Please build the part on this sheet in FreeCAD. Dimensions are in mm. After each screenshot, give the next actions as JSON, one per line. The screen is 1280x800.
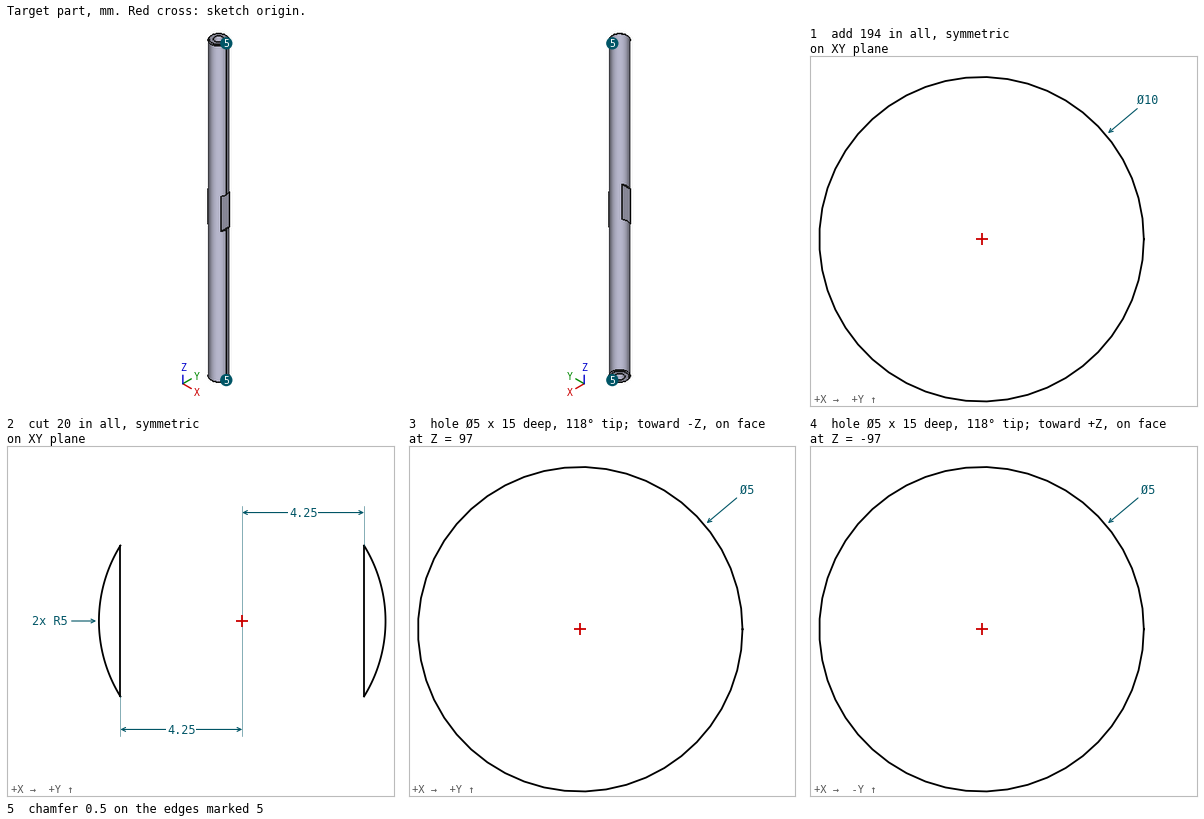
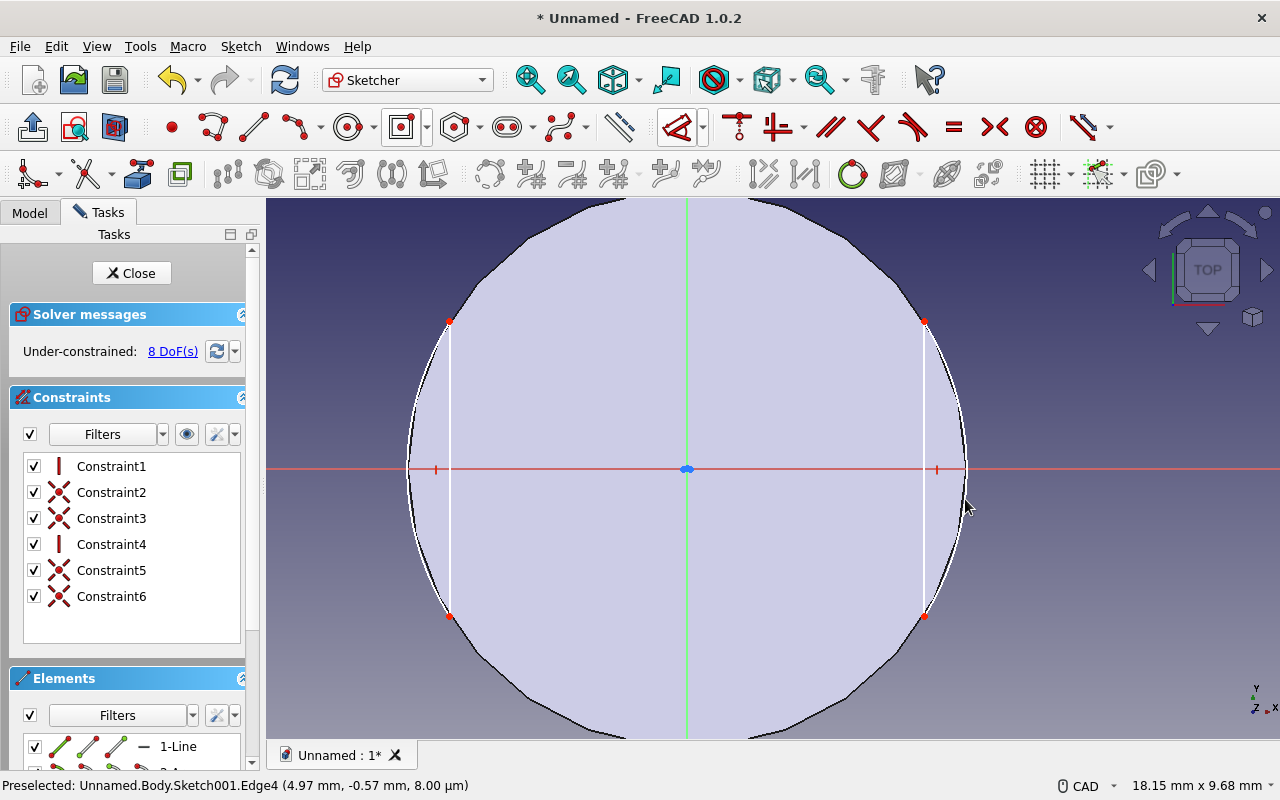
{"action": "left_click", "coordinate": [414, 408]}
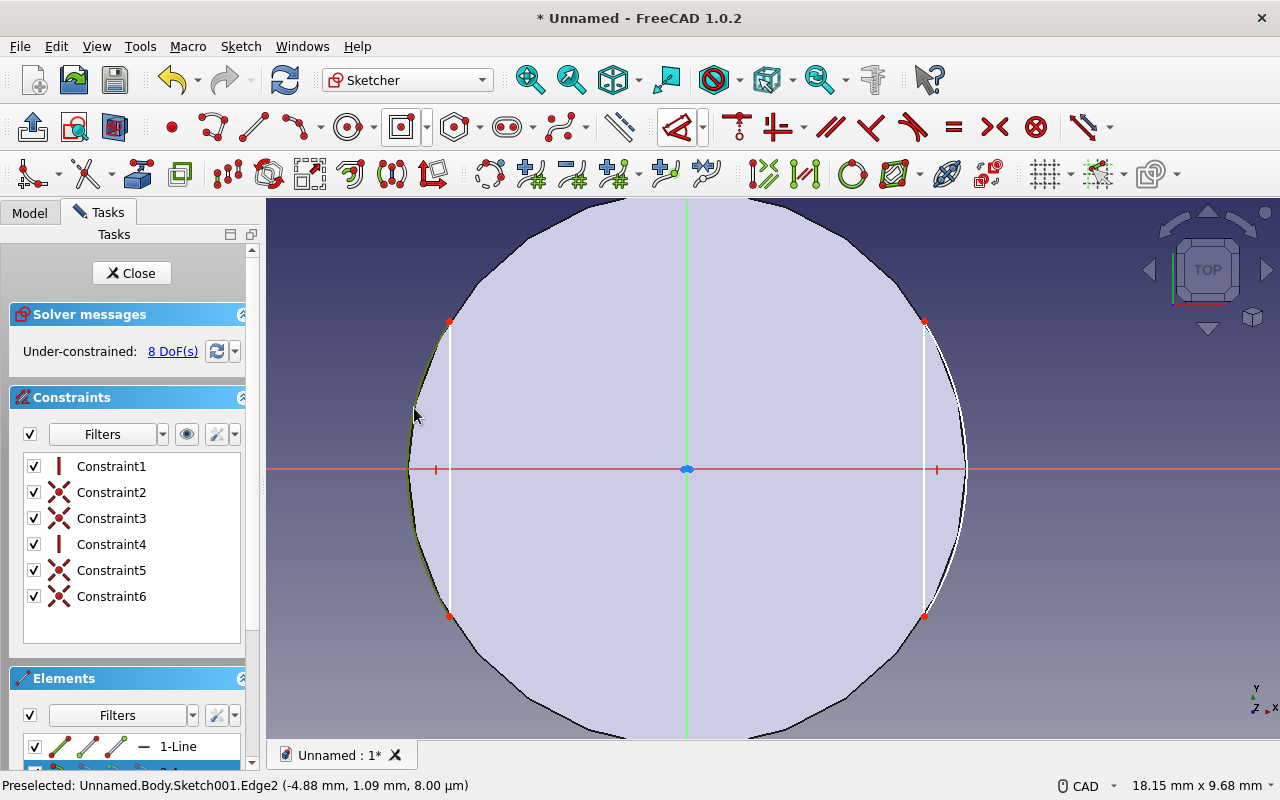
{"action": "left_click", "coordinate": [960, 531]}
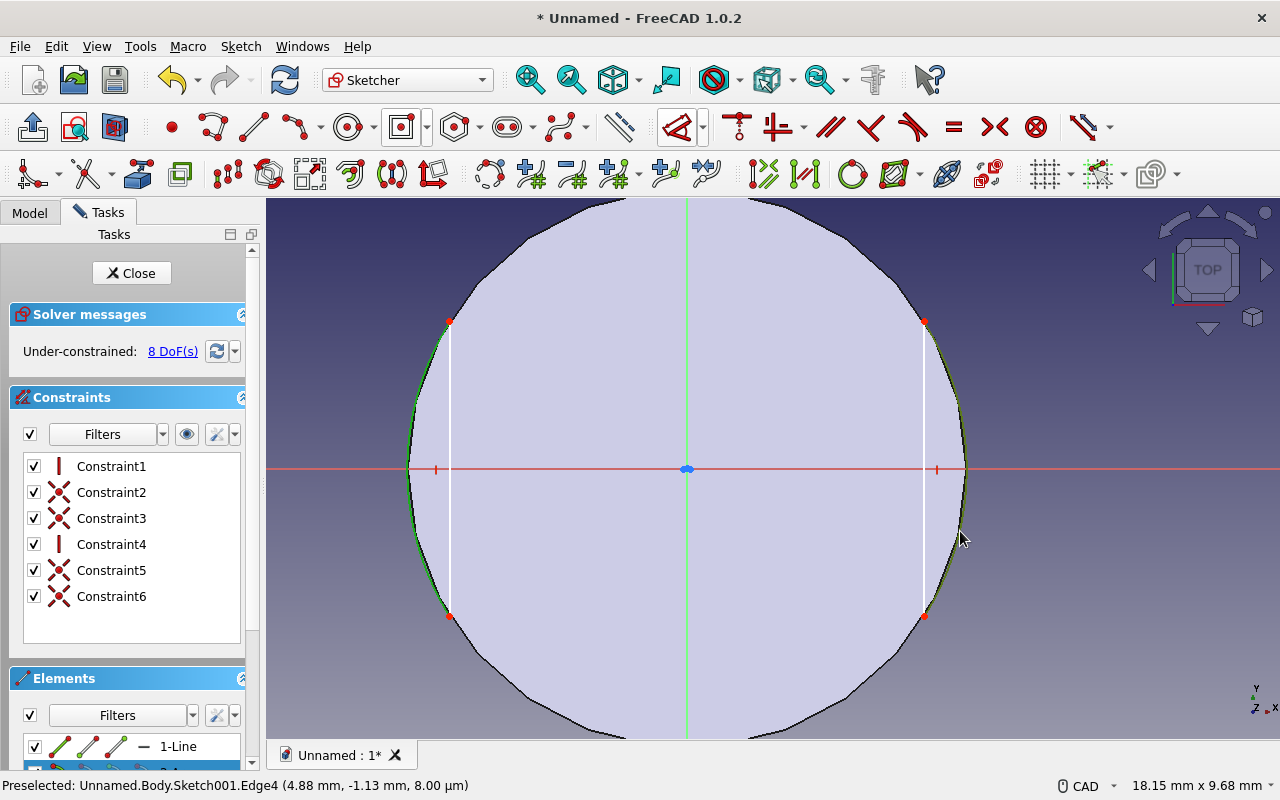
{"action": "left_click", "coordinate": [737, 128]}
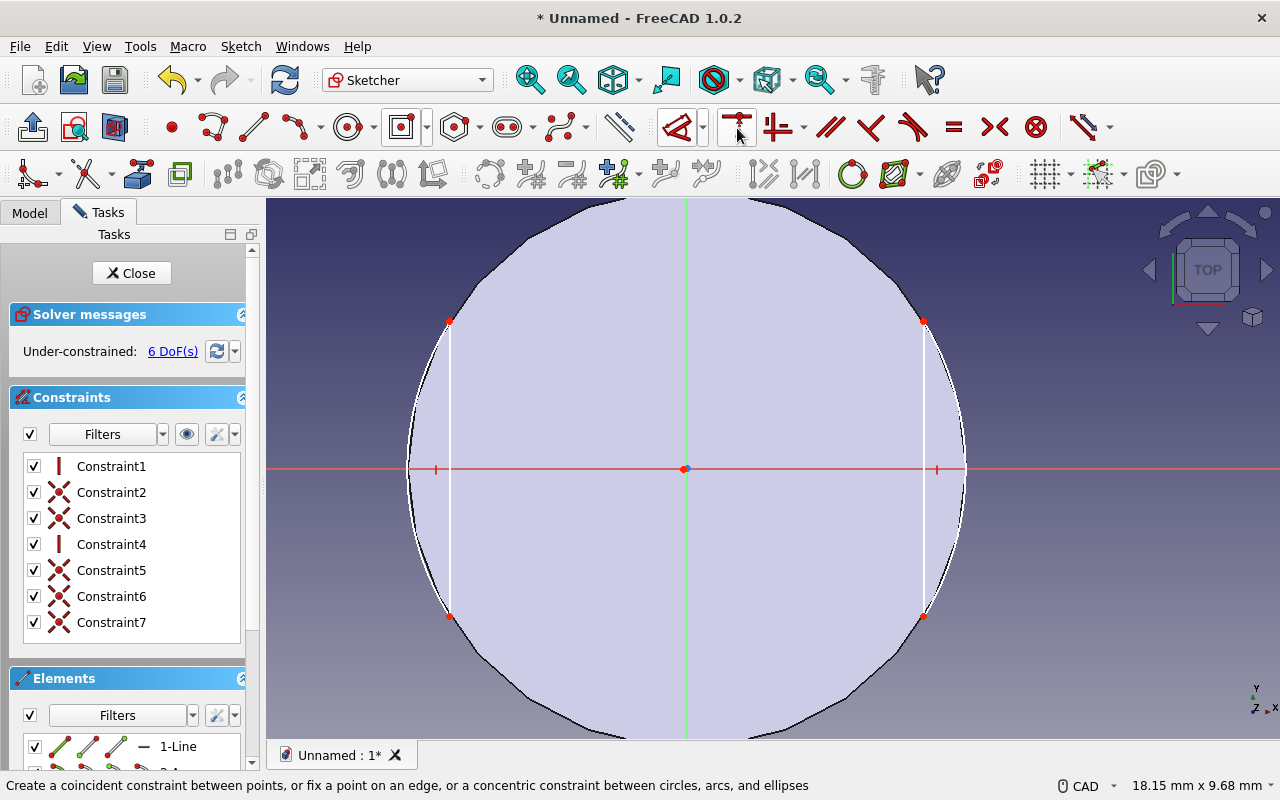
{"action": "left_click_drag", "start_coordinate": [674, 458], "coordinate": [697, 479]}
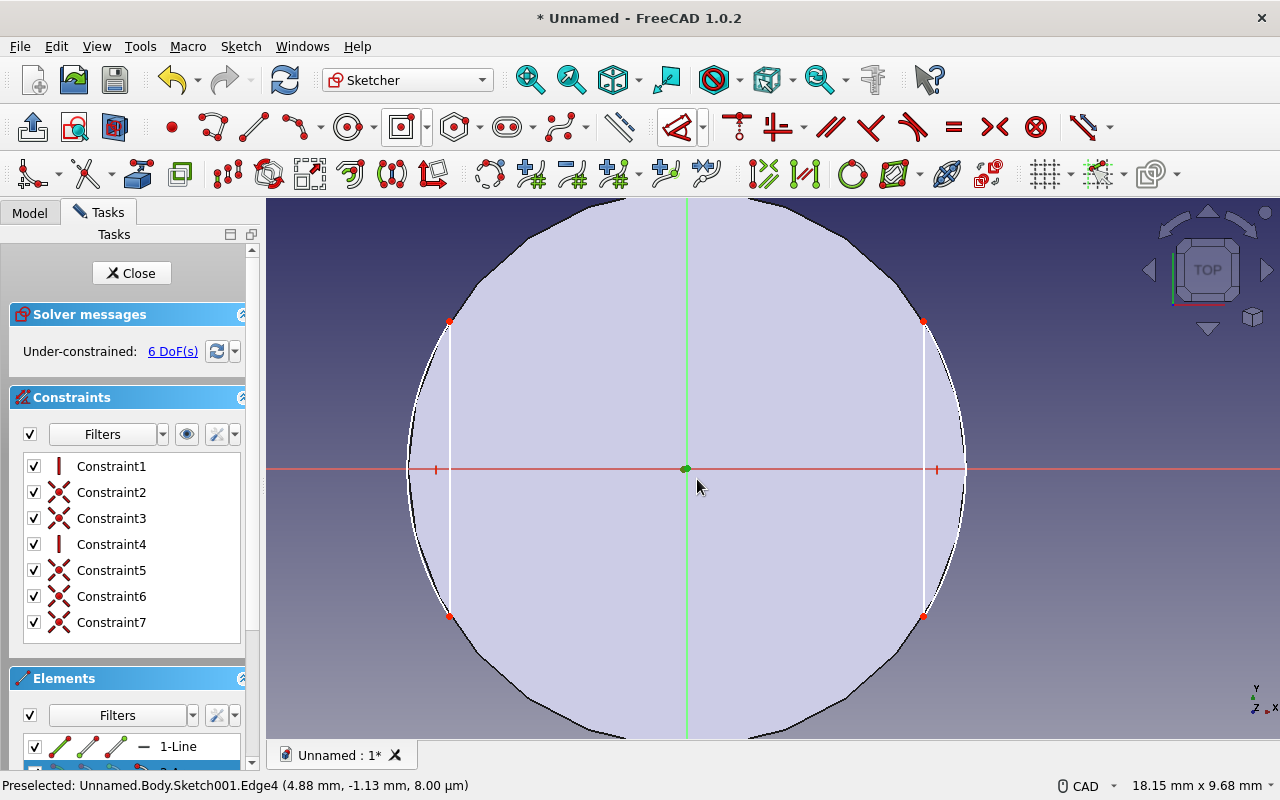
{"action": "left_click", "coordinate": [737, 128]}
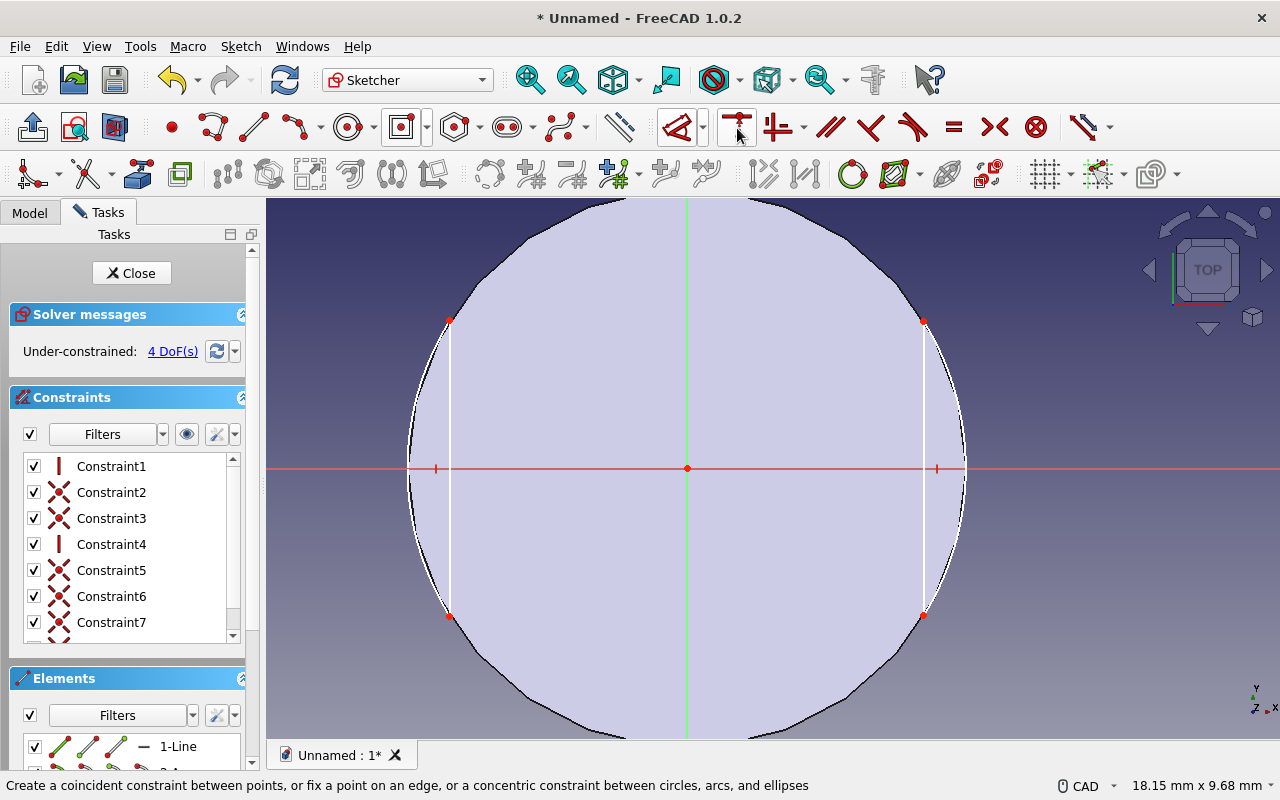
{"action": "left_click", "coordinate": [414, 407]}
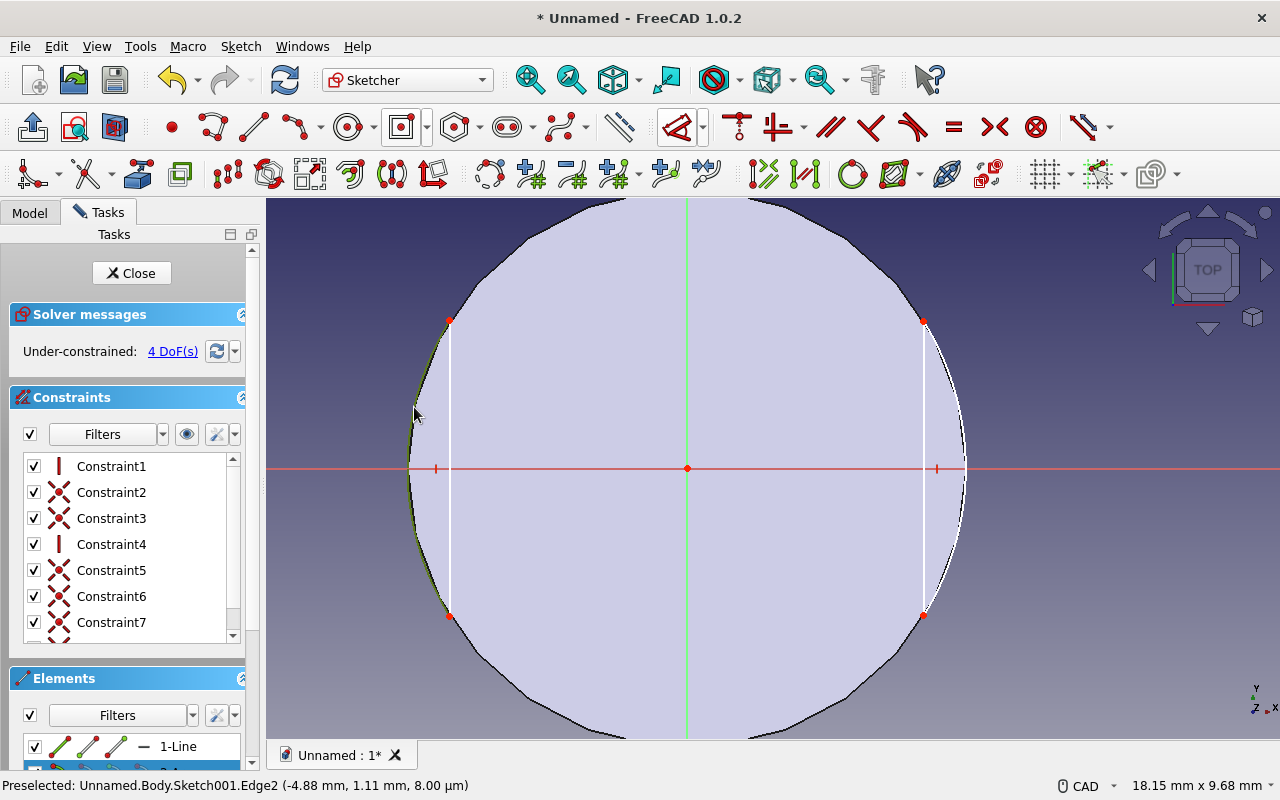
{"action": "left_click", "coordinate": [959, 530]}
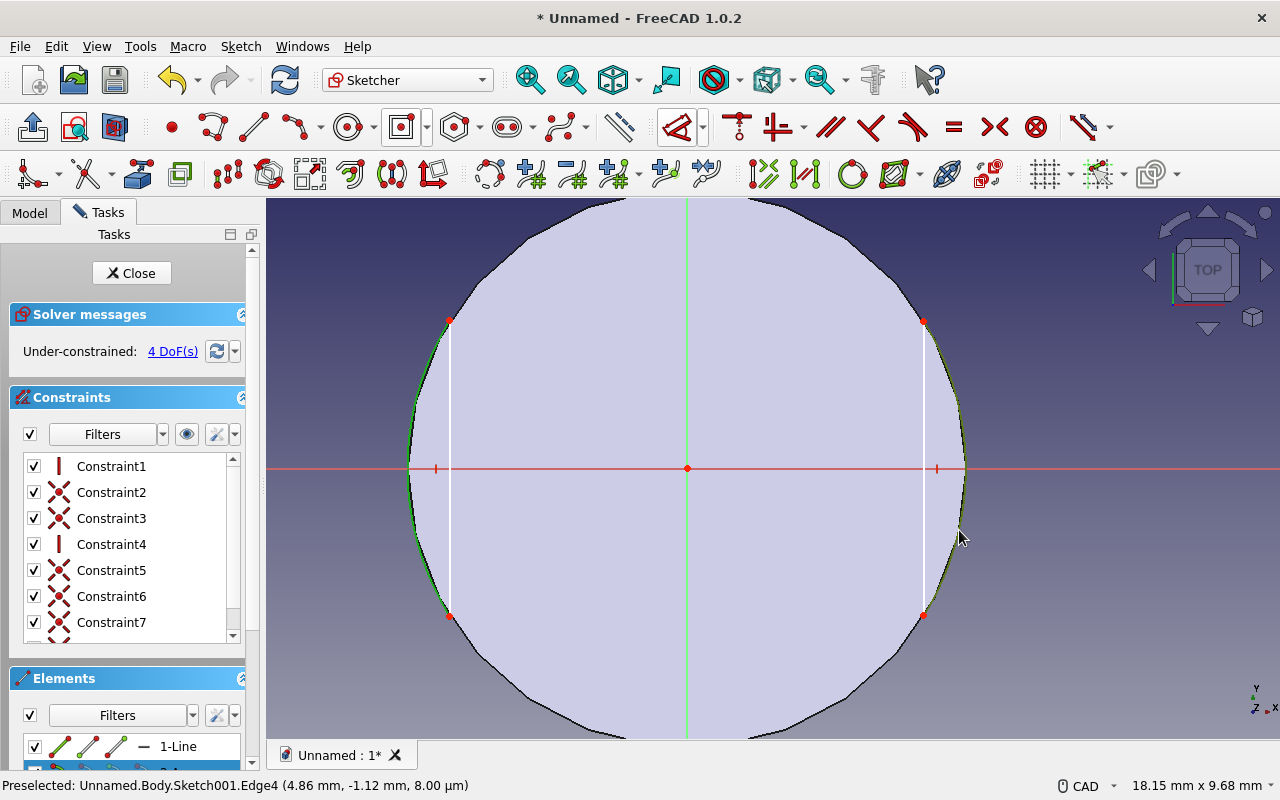
{"action": "left_click", "coordinate": [954, 128]}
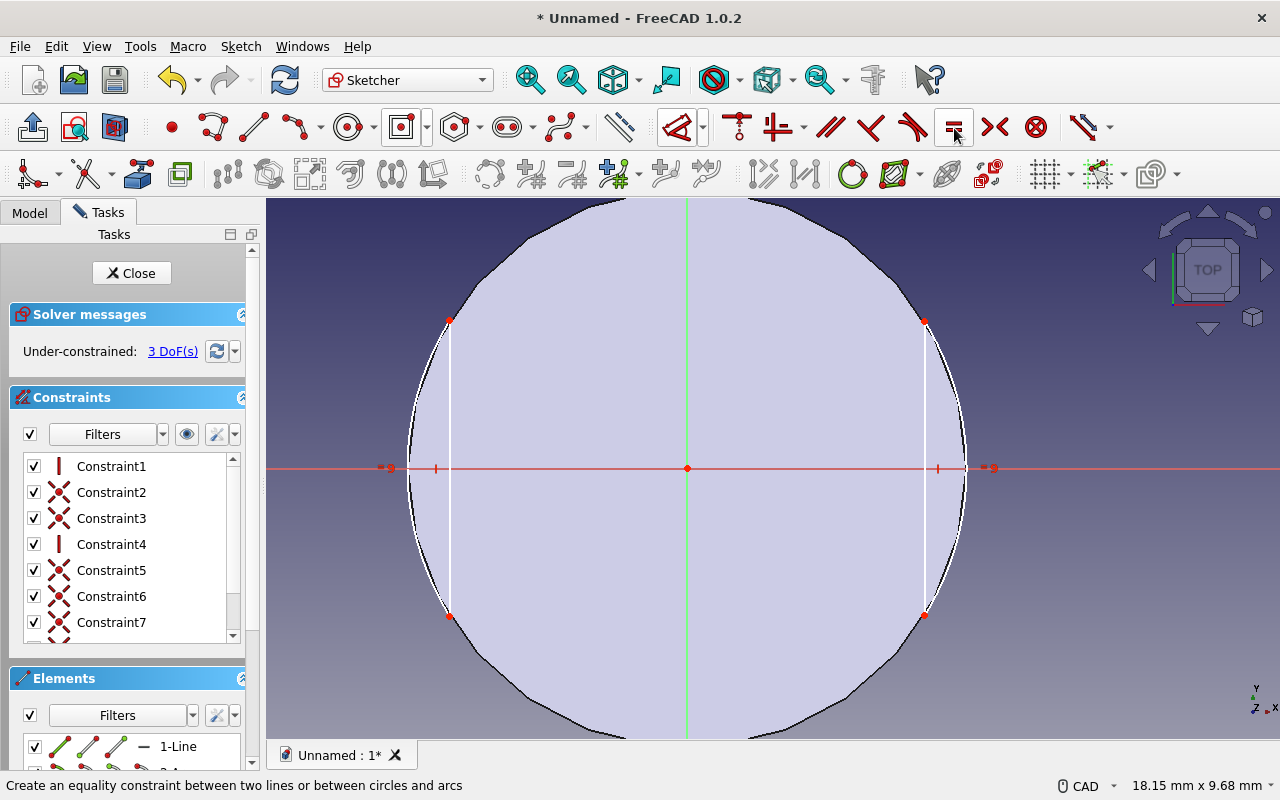
{"action": "left_click", "coordinate": [414, 407]}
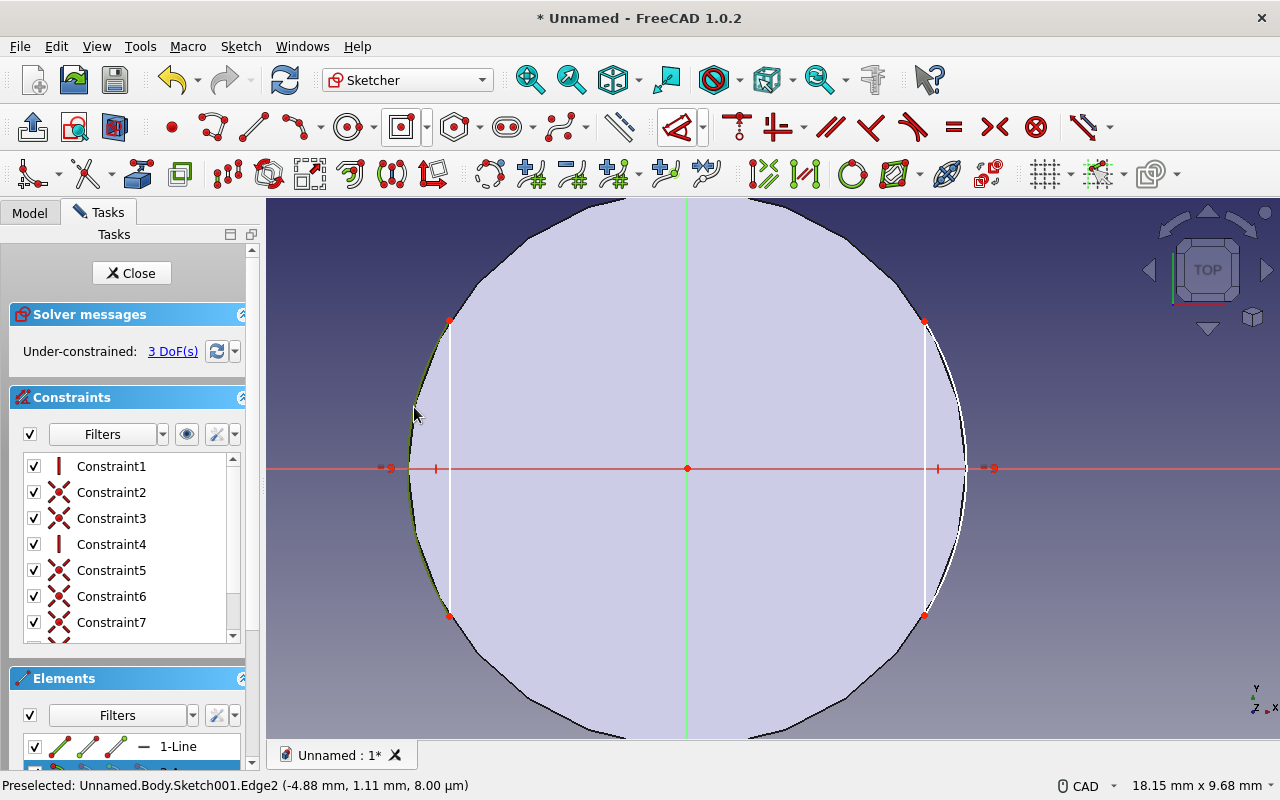
{"action": "left_click", "coordinate": [702, 128]}